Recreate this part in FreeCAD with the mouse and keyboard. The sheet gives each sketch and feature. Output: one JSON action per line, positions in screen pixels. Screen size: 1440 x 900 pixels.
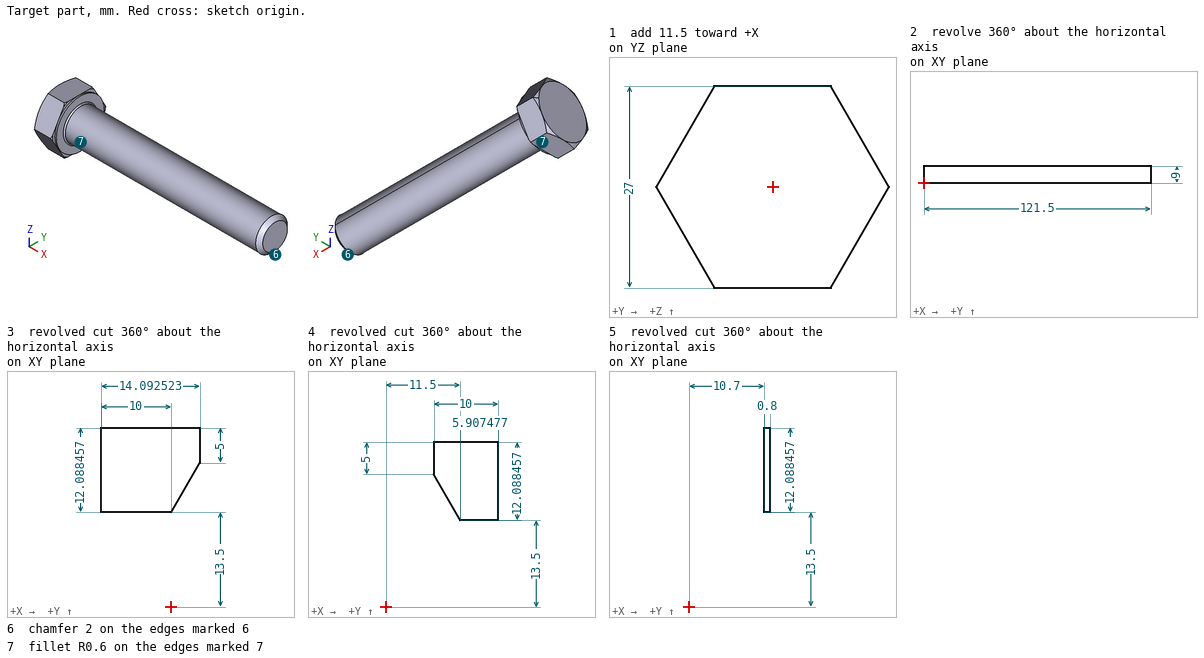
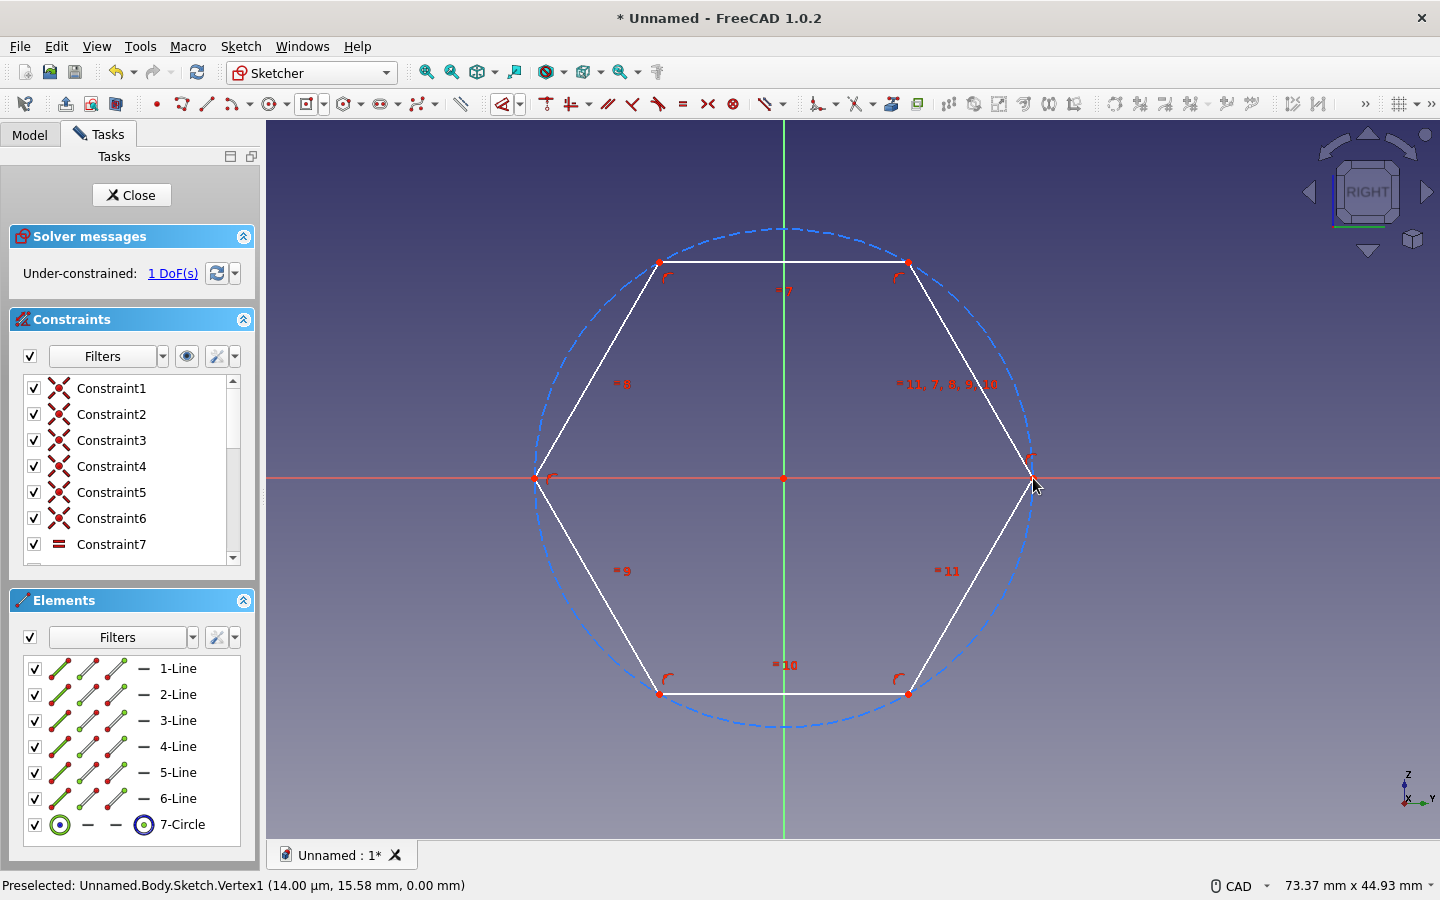
{"action": "left_click", "coordinate": [502, 104]}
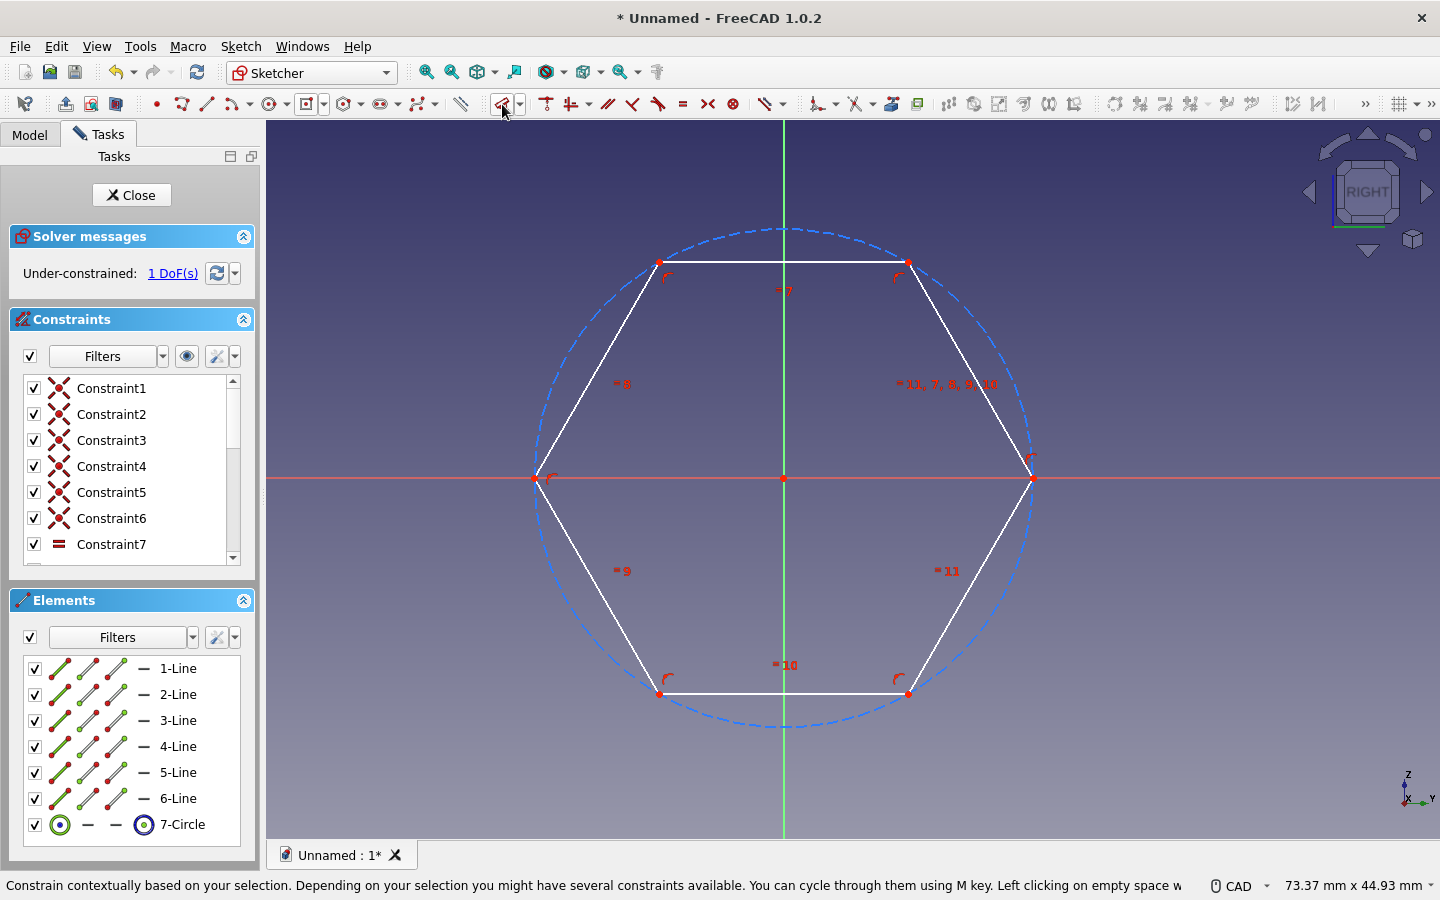
{"action": "left_click", "coordinate": [659, 694]}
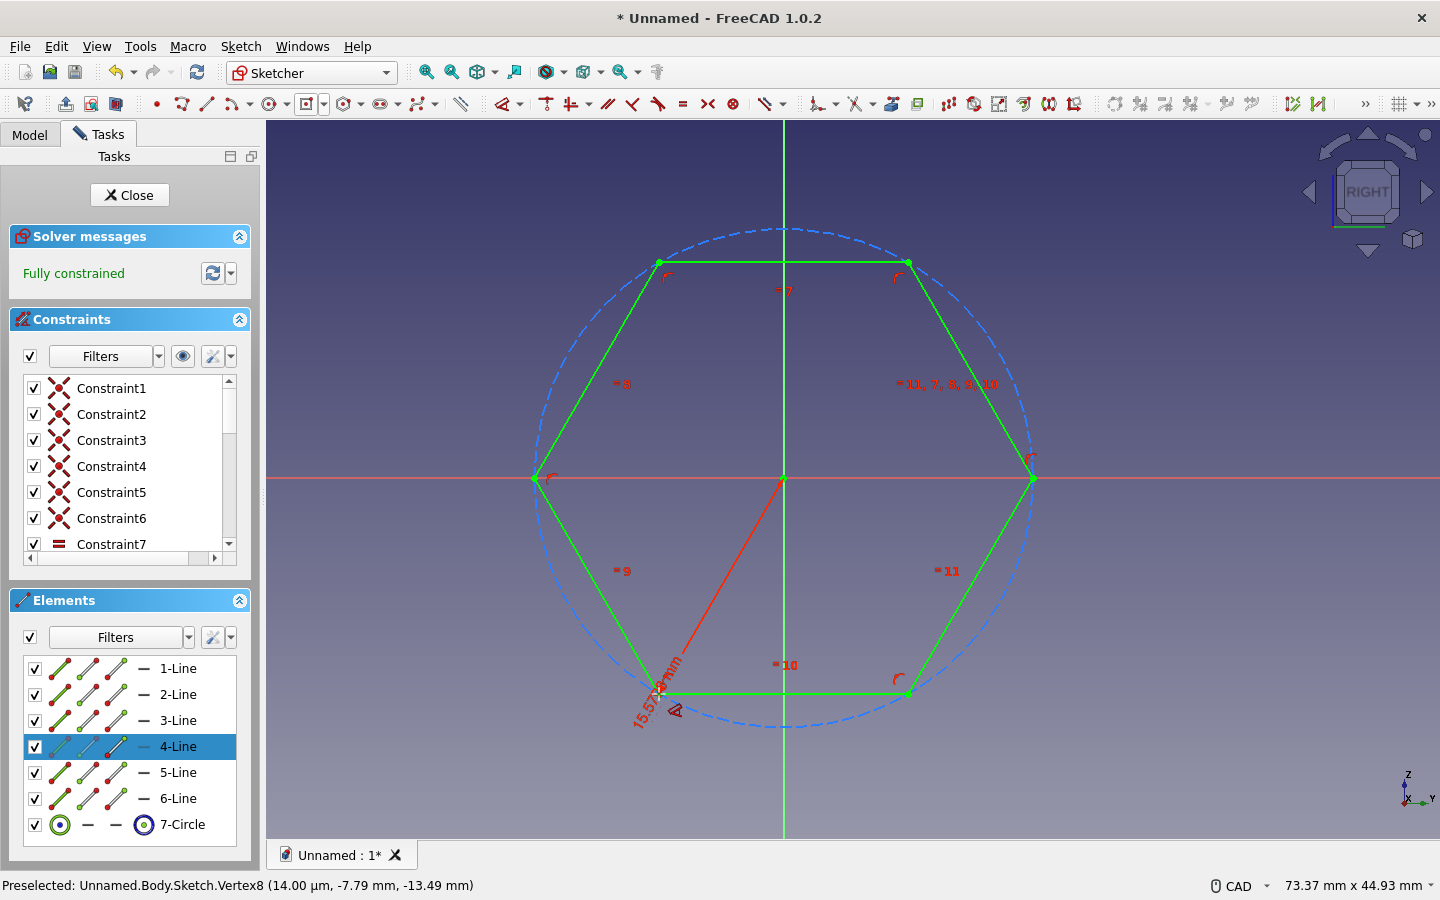
{"action": "left_click", "coordinate": [908, 262]}
{"action": "left_click", "coordinate": [625, 379]}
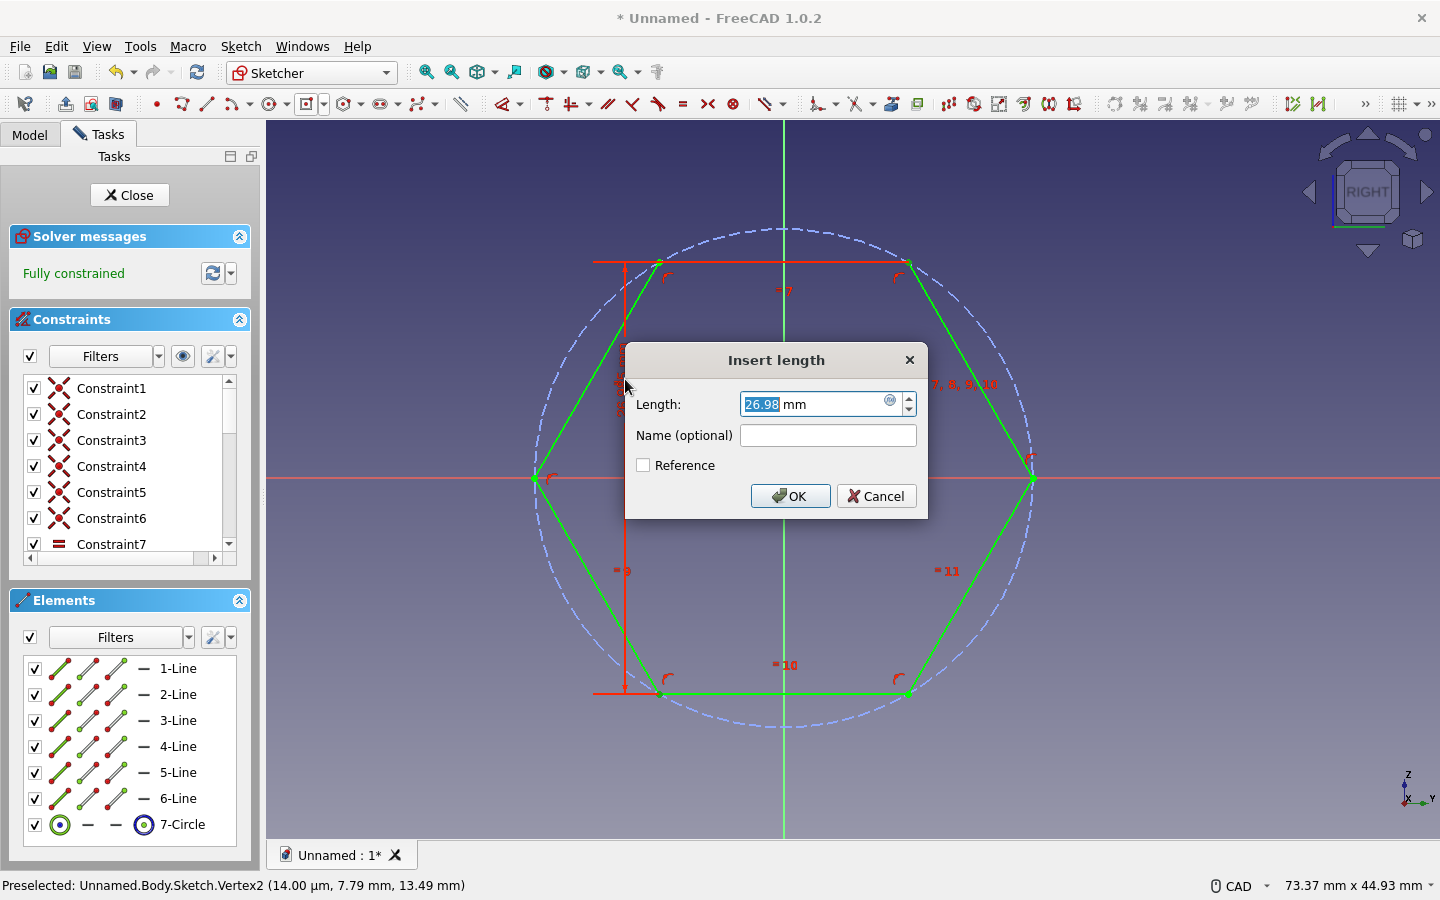
{"action": "type", "text": "27"}
{"action": "key", "text": "Return"}
{"action": "key", "text": "Escape"}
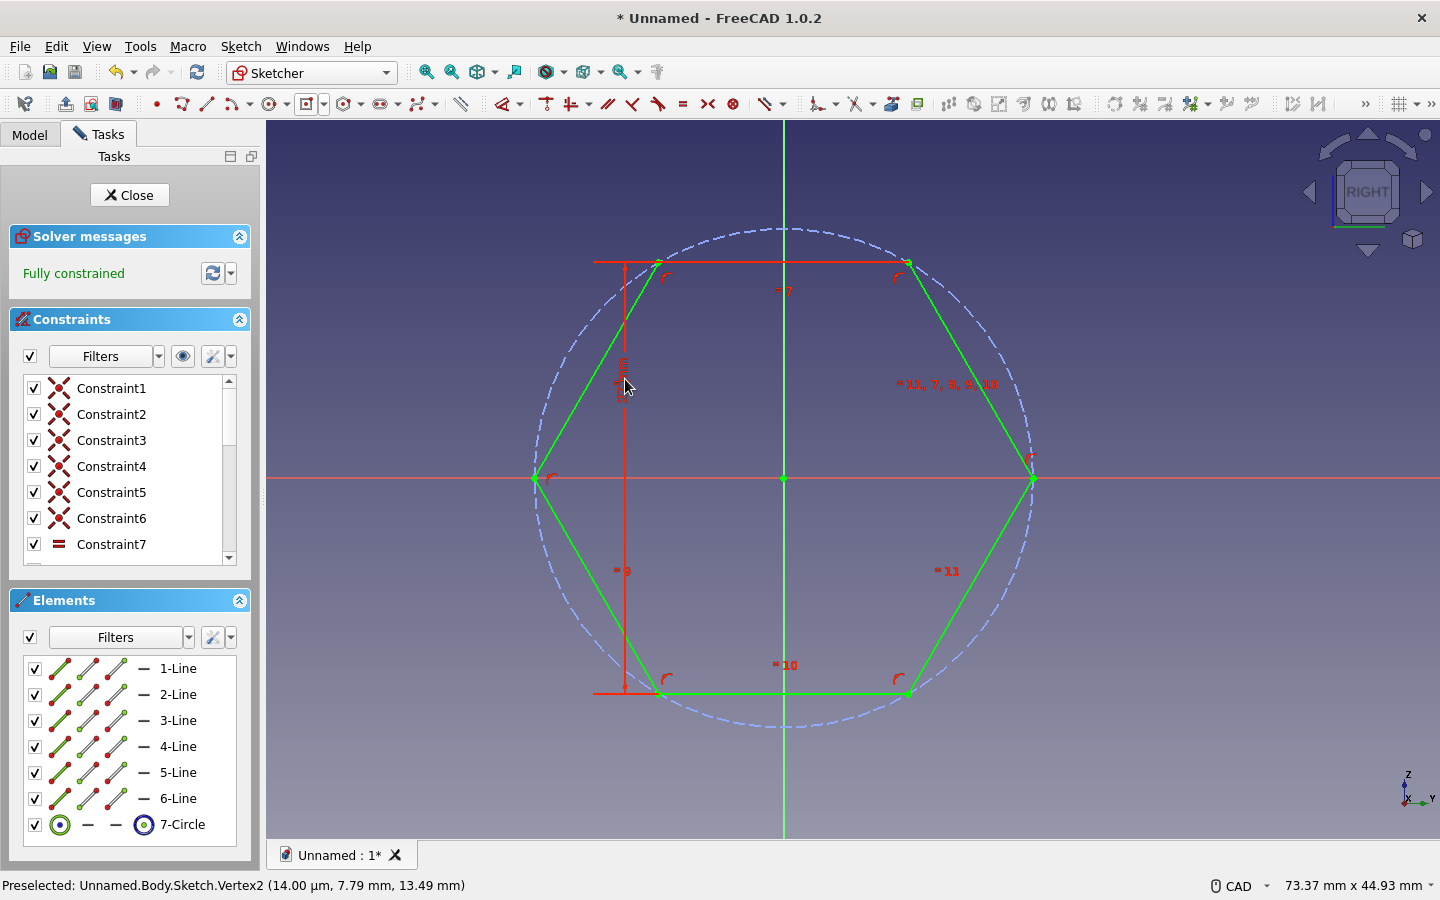
{"action": "left_click", "coordinate": [130, 195]}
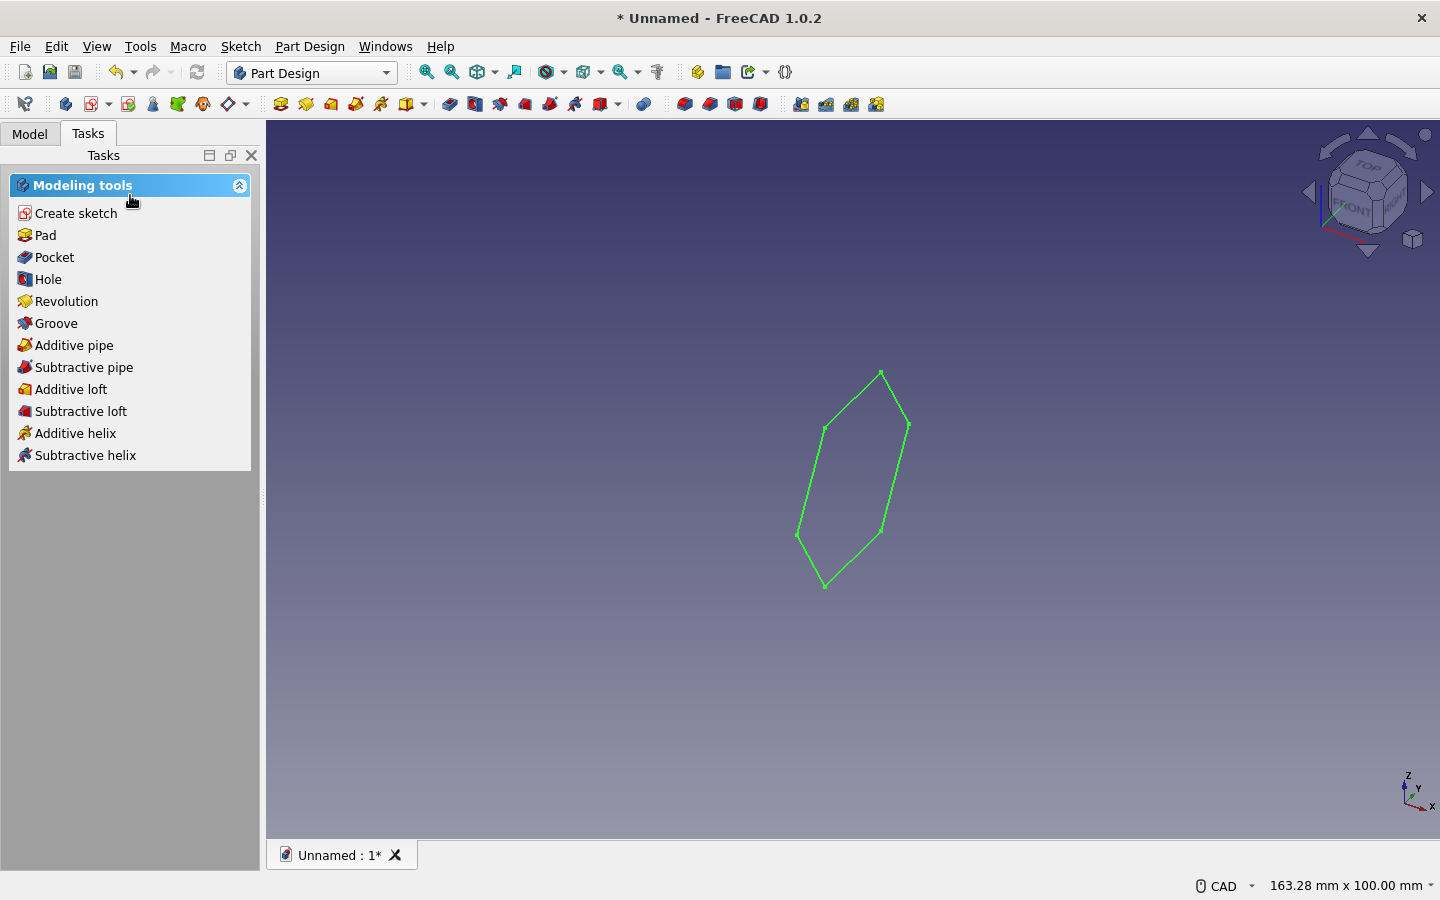
{"action": "left_click", "coordinate": [281, 104]}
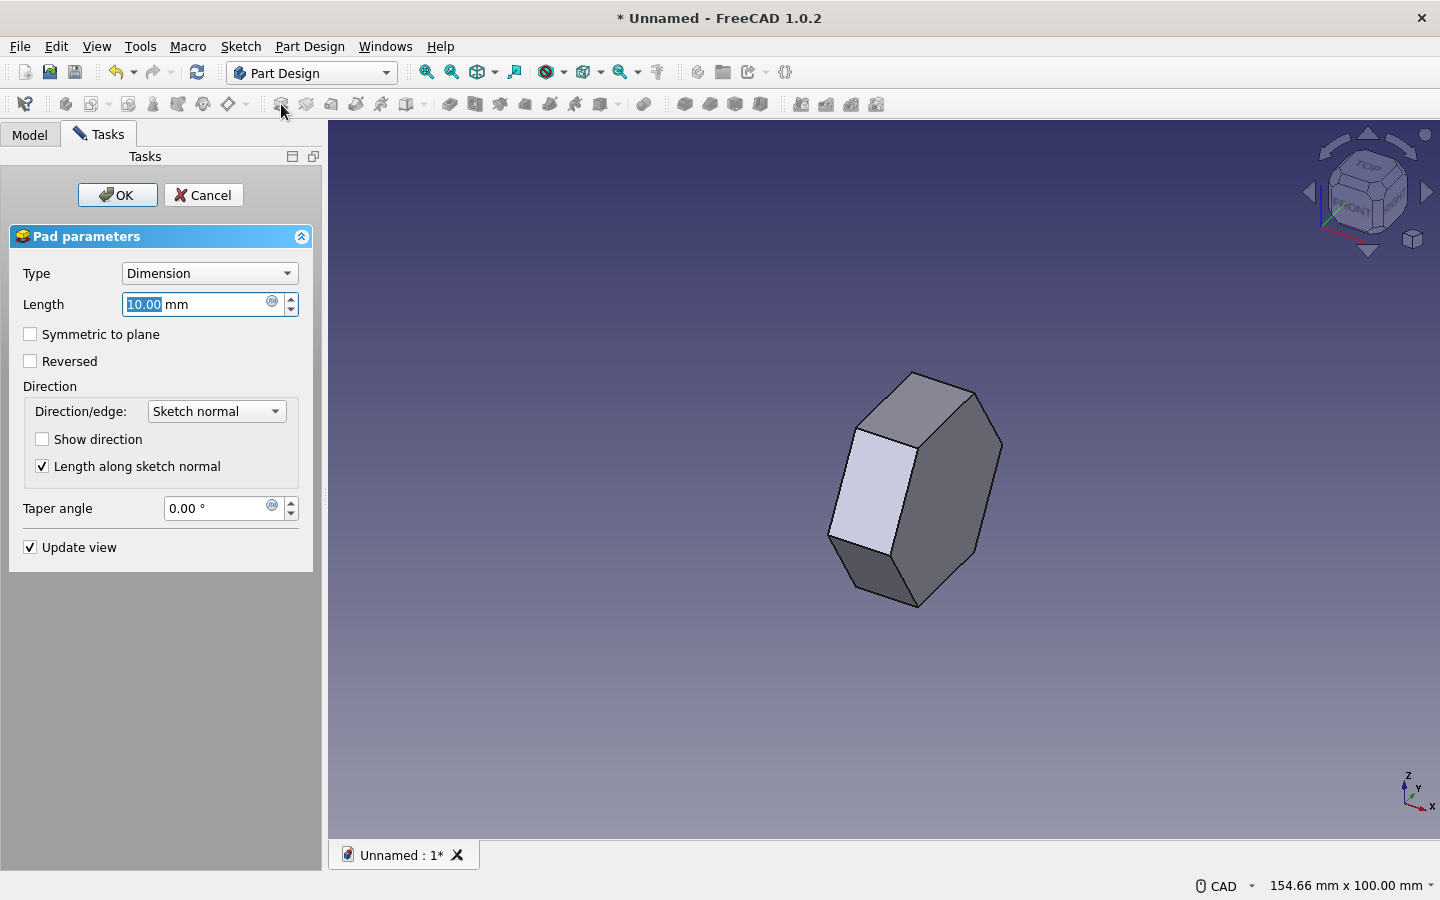
{"action": "type", "text": "11.5"}
{"action": "key", "text": "Tab"}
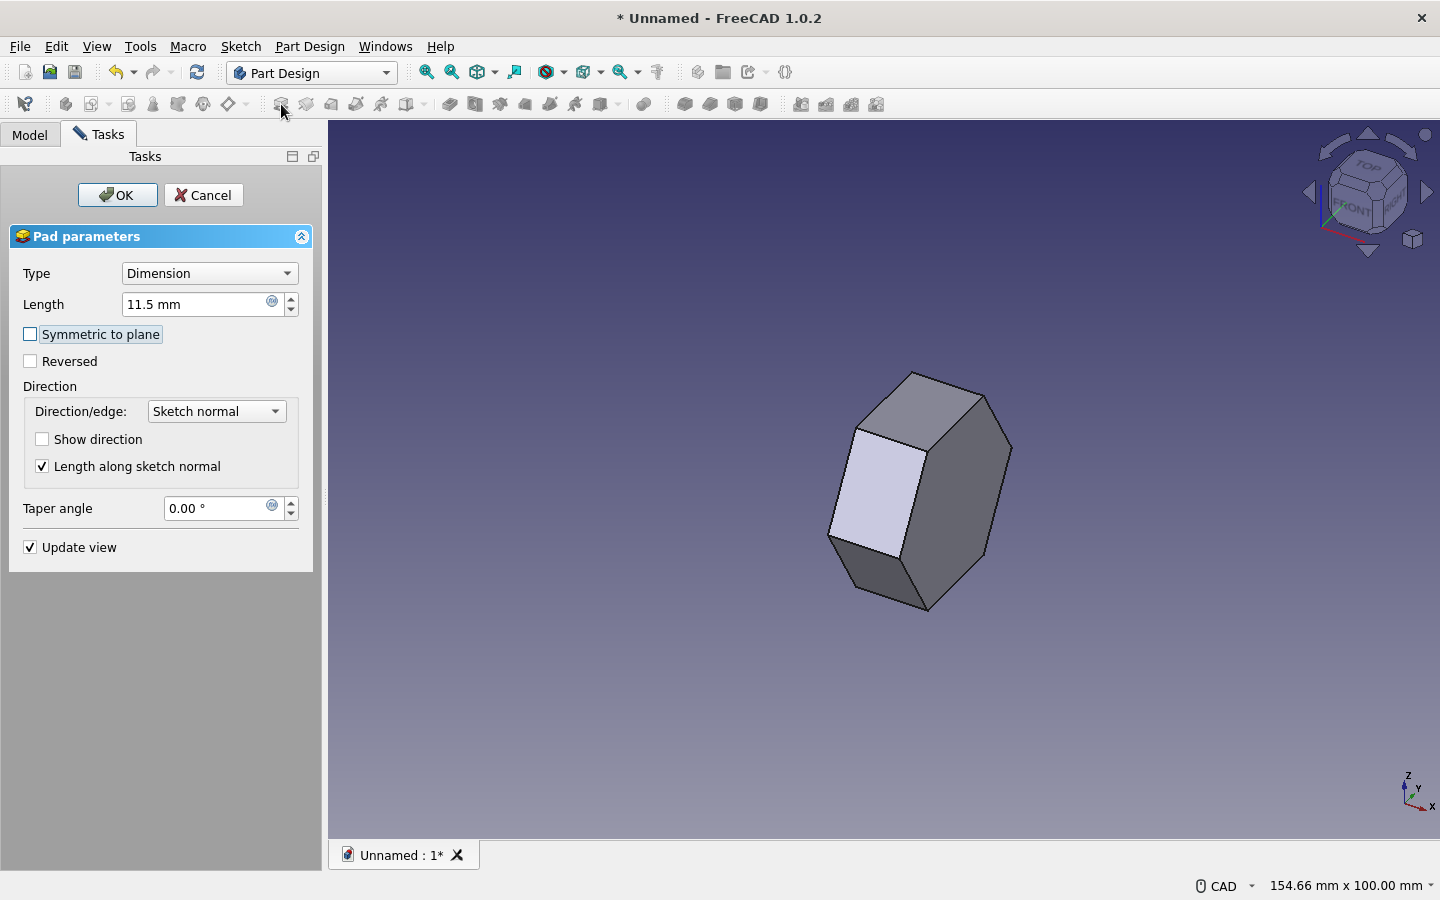
{"action": "left_click", "coordinate": [118, 195]}